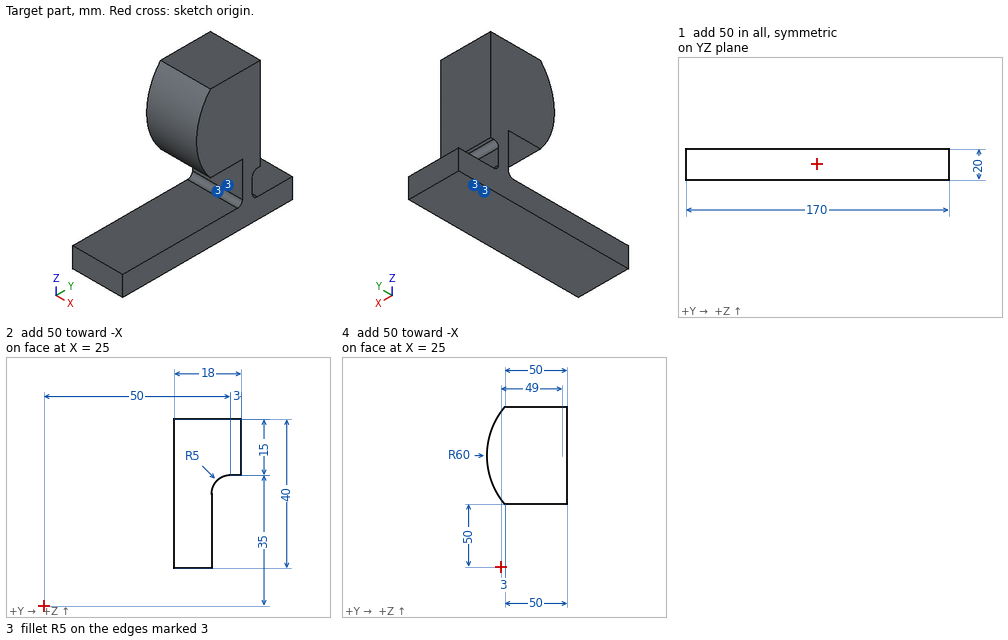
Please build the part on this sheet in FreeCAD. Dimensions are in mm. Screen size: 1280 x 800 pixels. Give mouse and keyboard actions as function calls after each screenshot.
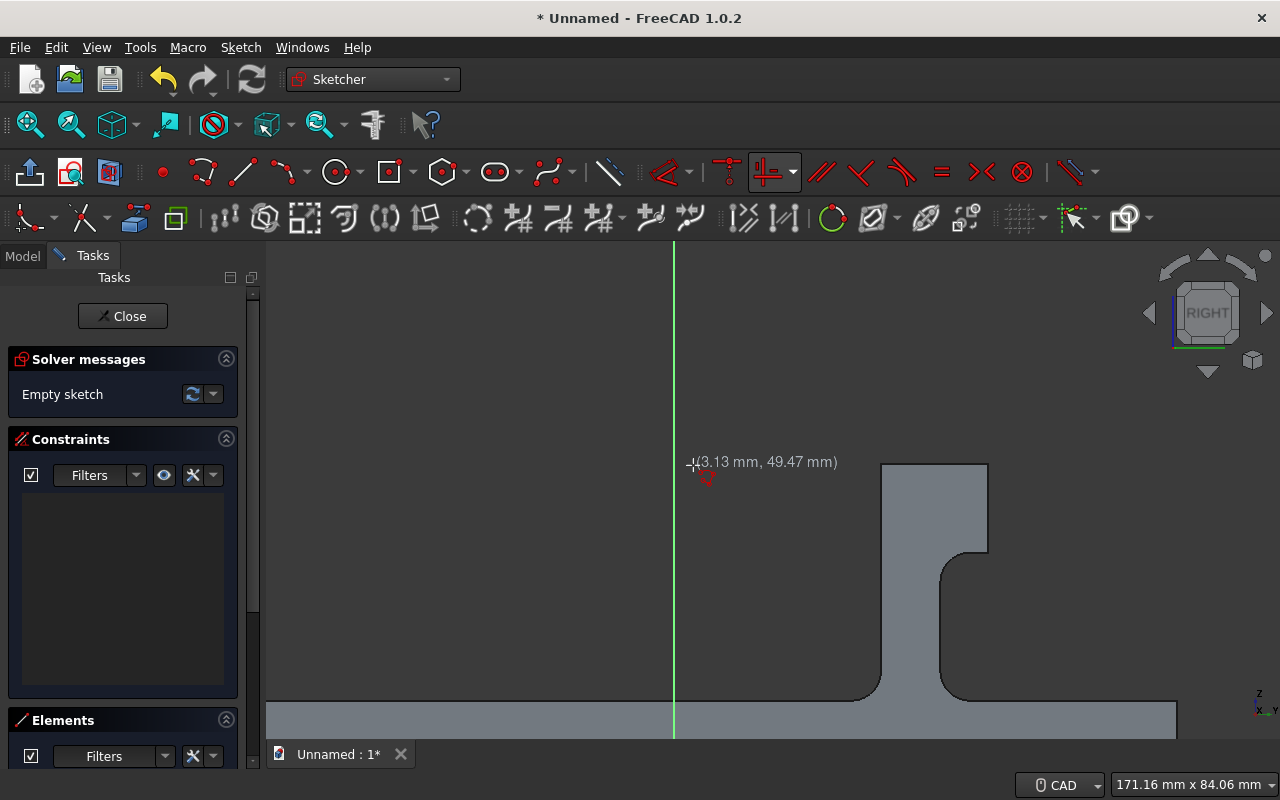
click(692, 464)
click(988, 464)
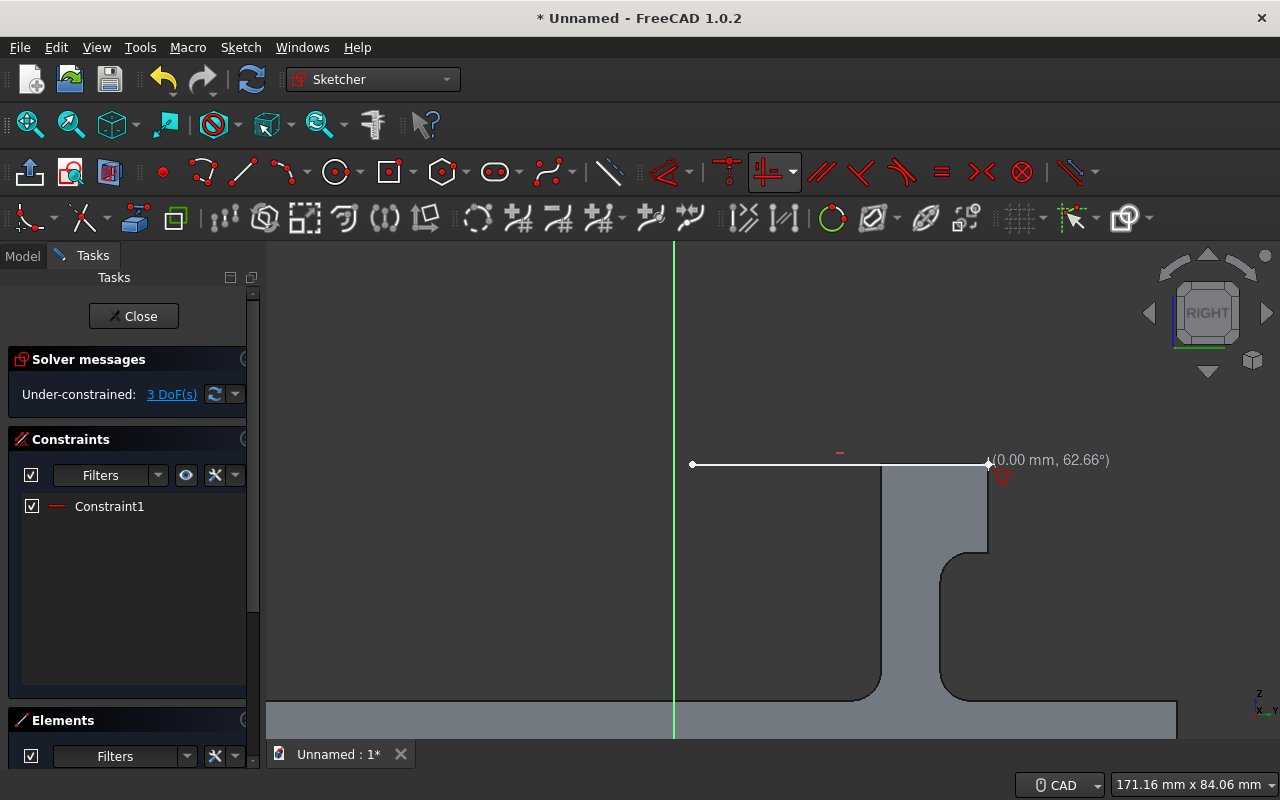
scroll(628, 577, down, 4)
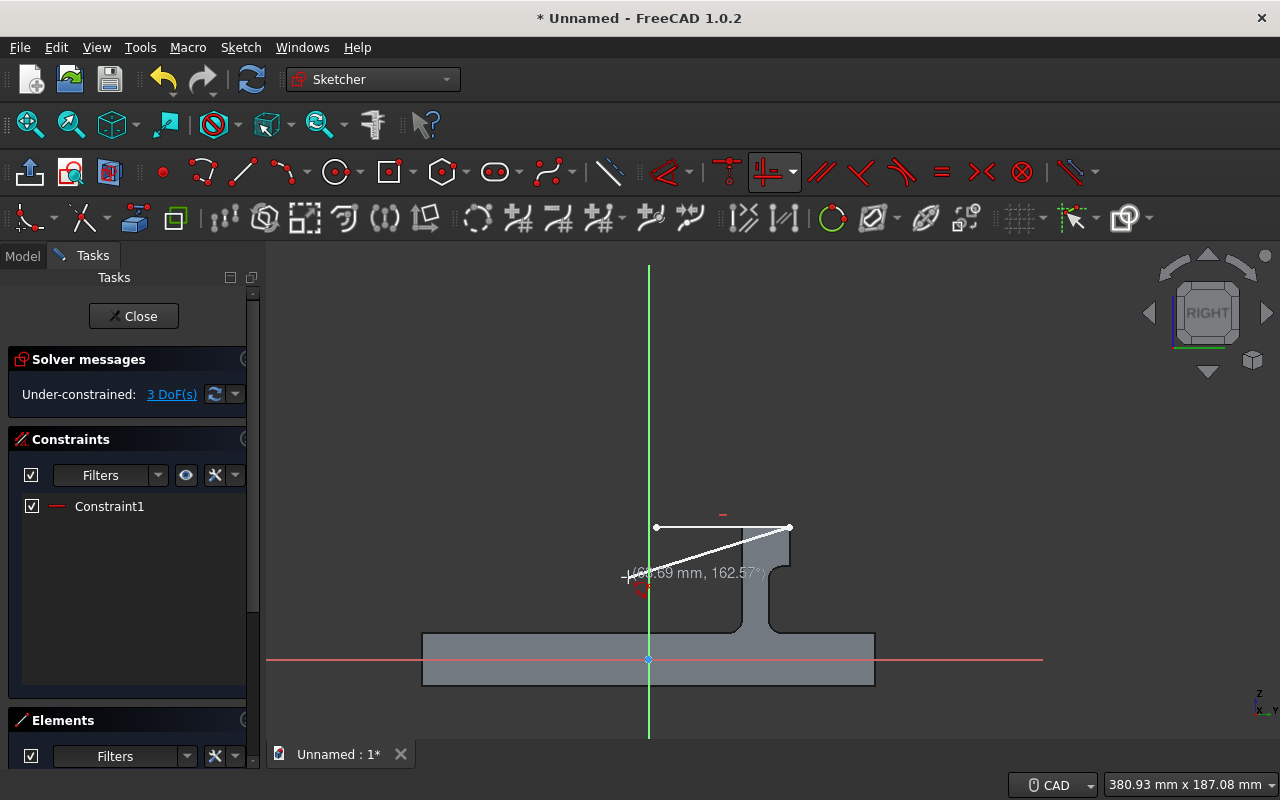
click(790, 321)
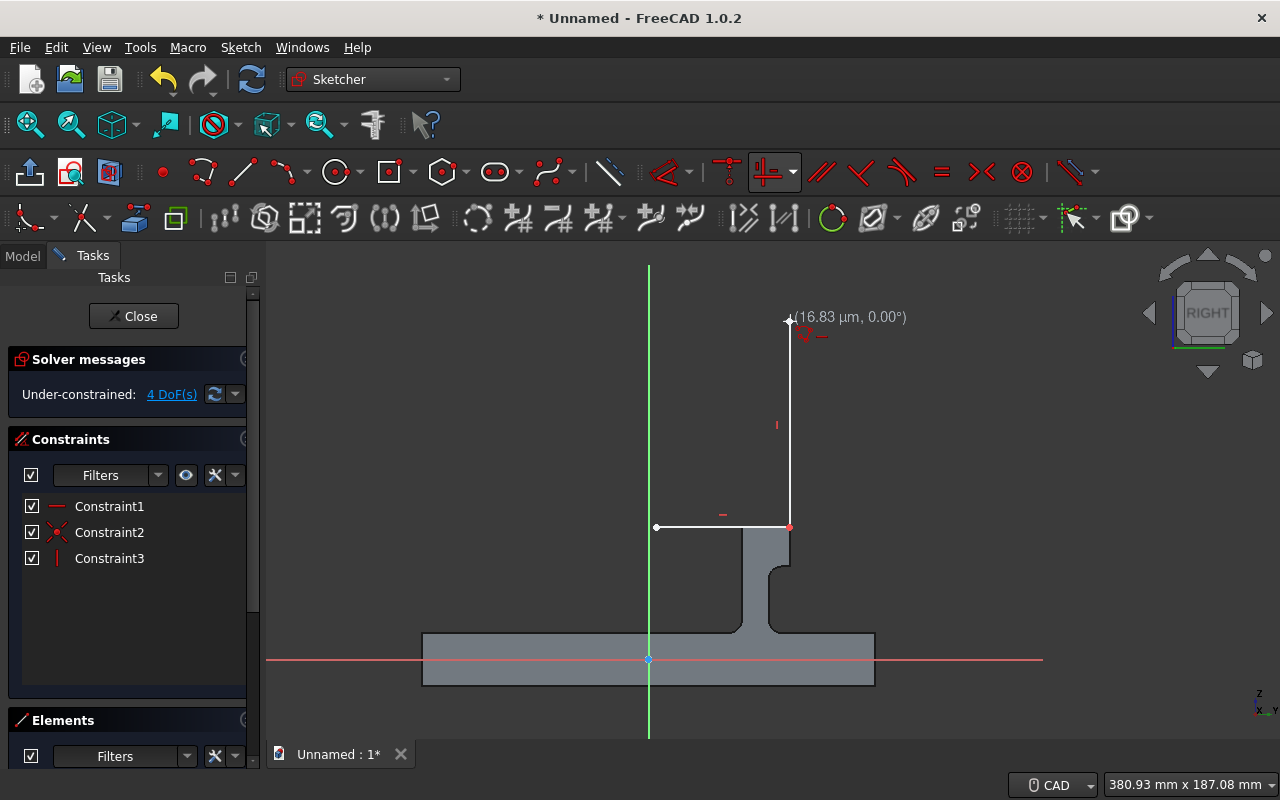
scroll(657, 321, up, 4)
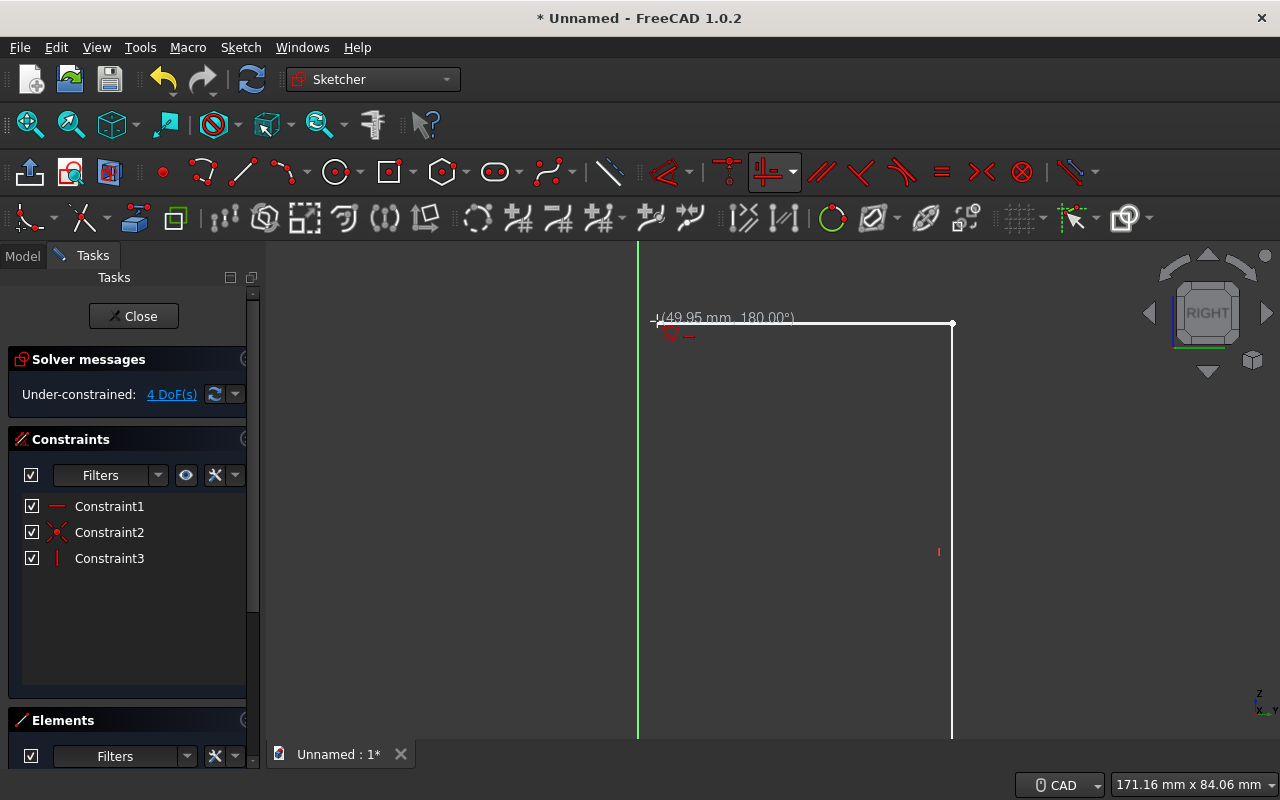
click(656, 321)
right_click(656, 321)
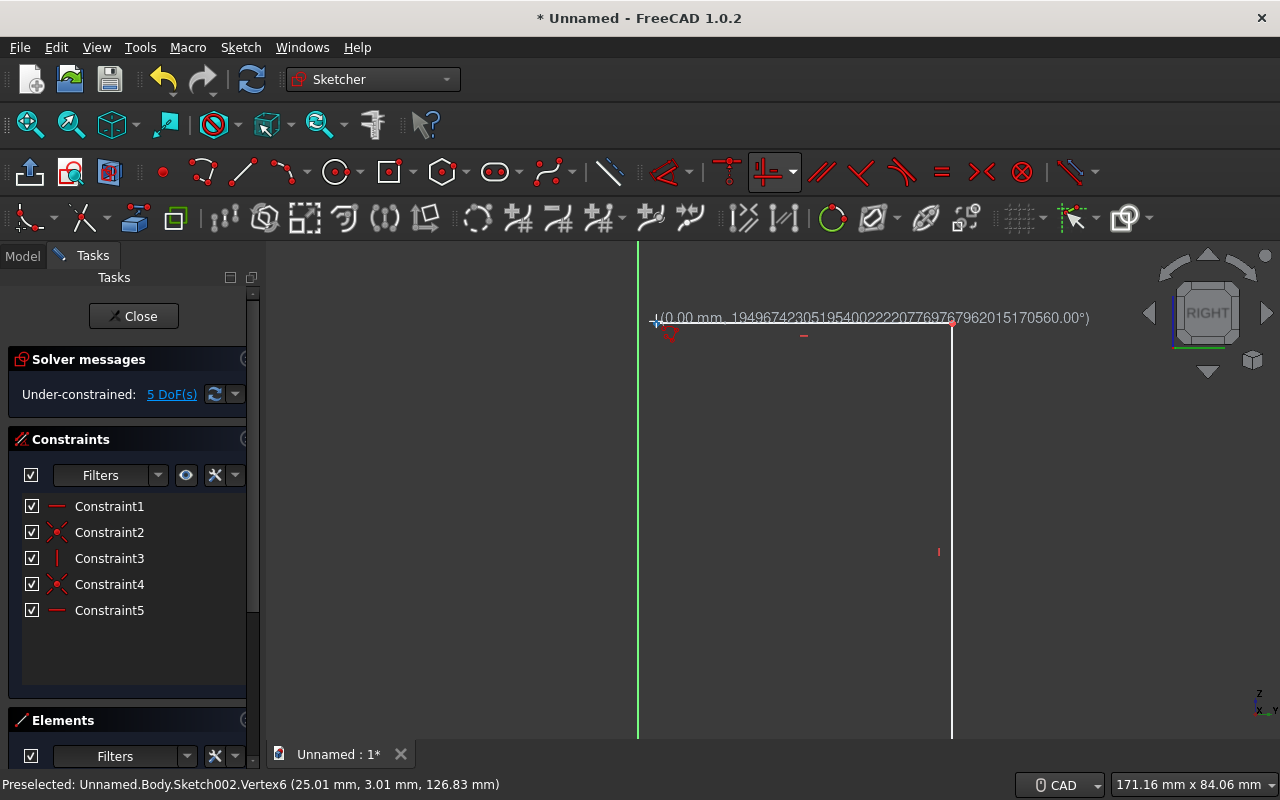
key(g)
key(3)
key(a)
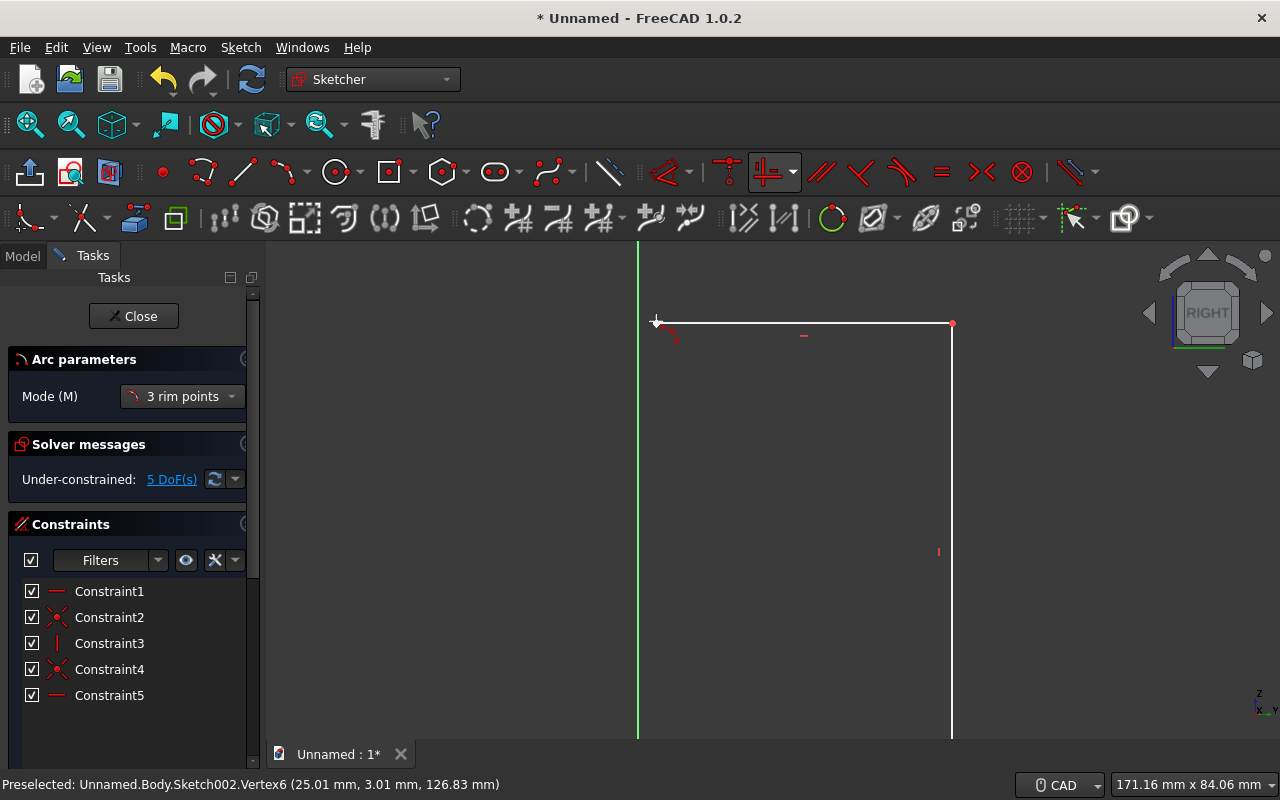
click(656, 323)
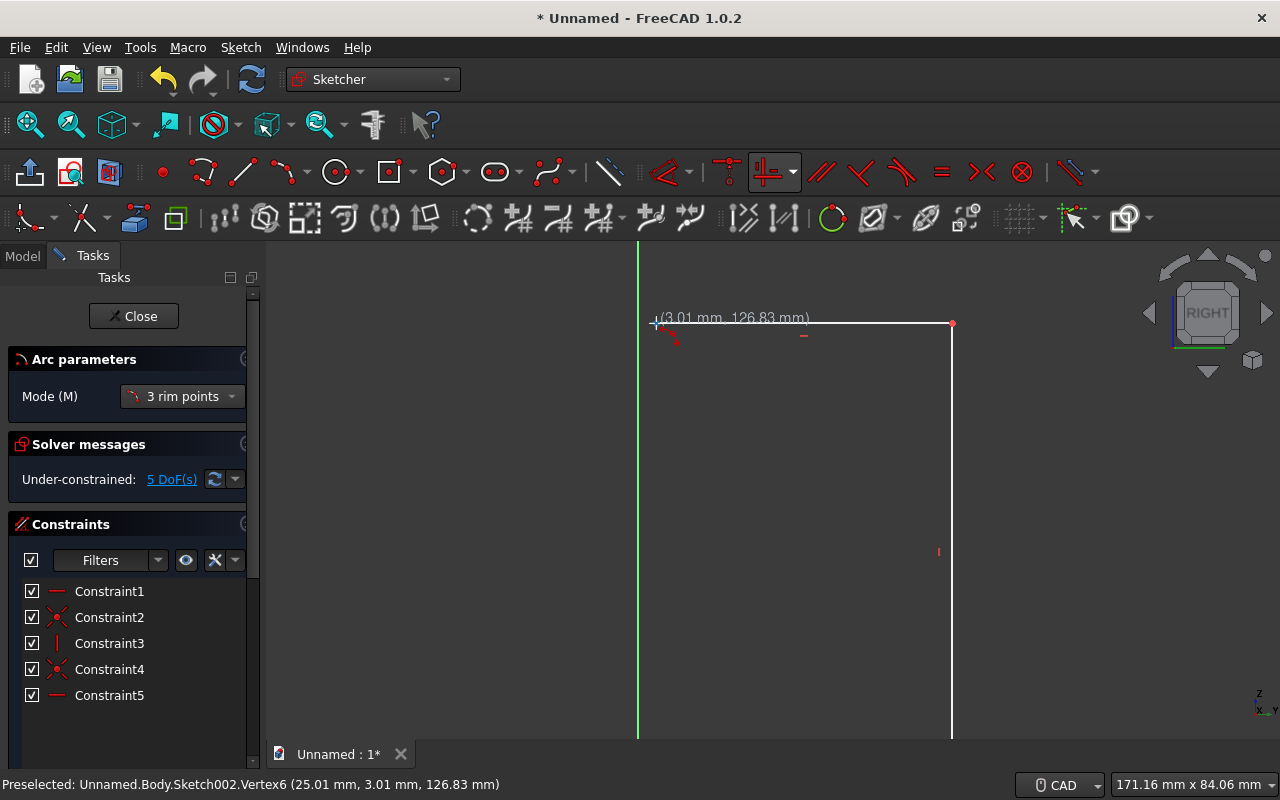
scroll(657, 320, down, 4)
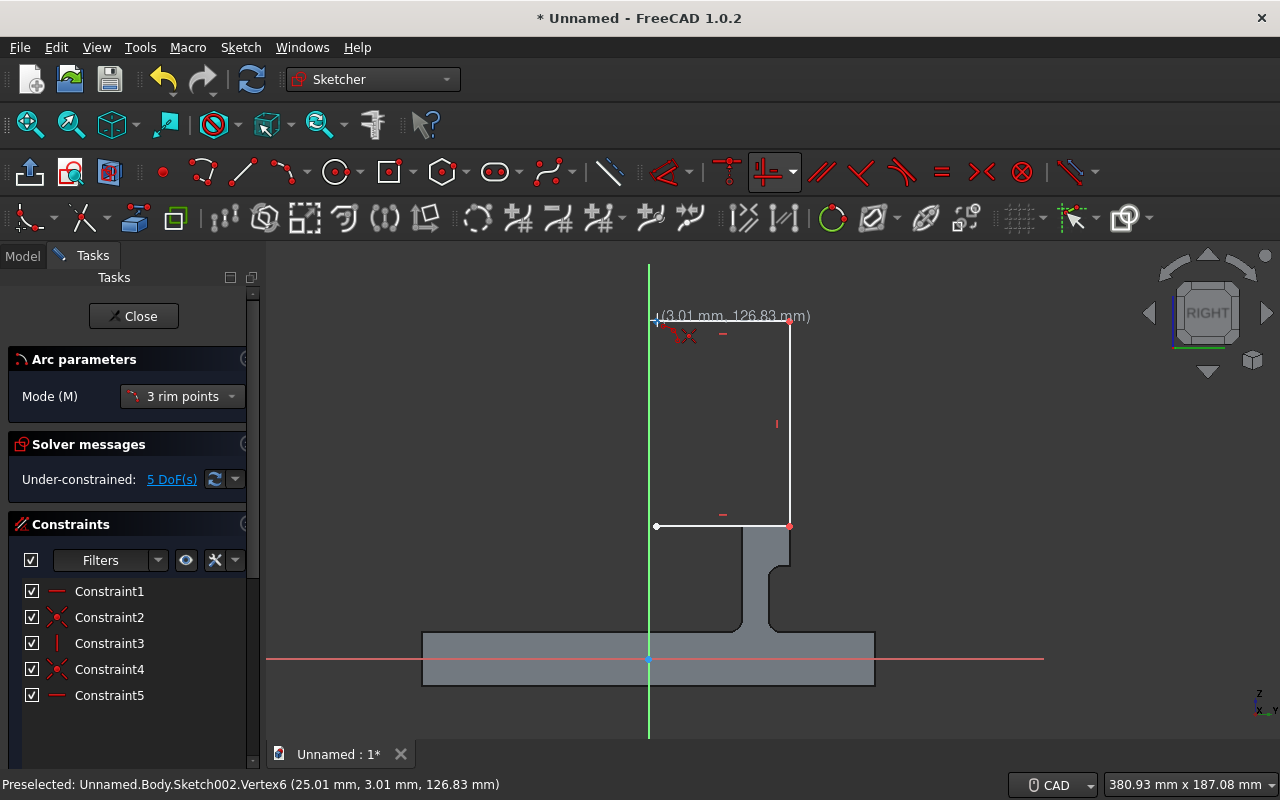
scroll(657, 526, up, 4)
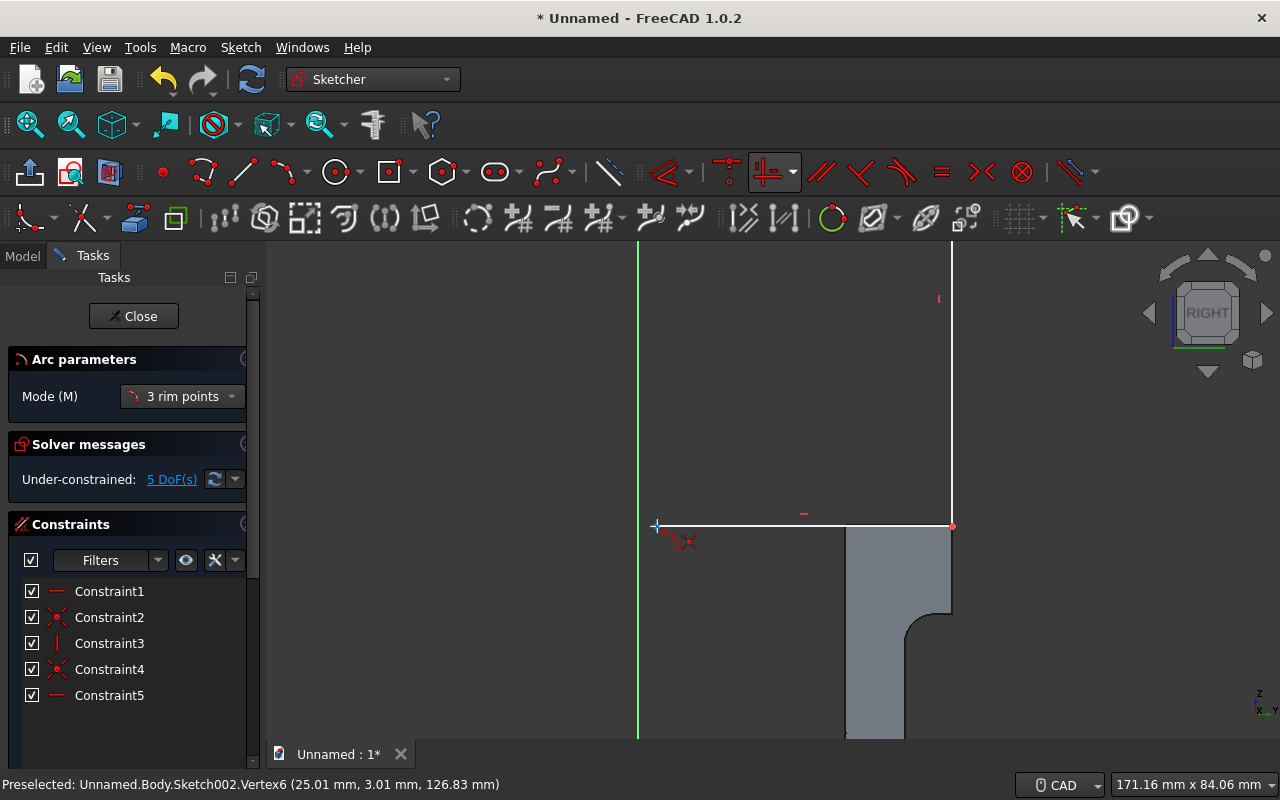
click(656, 526)
click(573, 297)
key(Escape)